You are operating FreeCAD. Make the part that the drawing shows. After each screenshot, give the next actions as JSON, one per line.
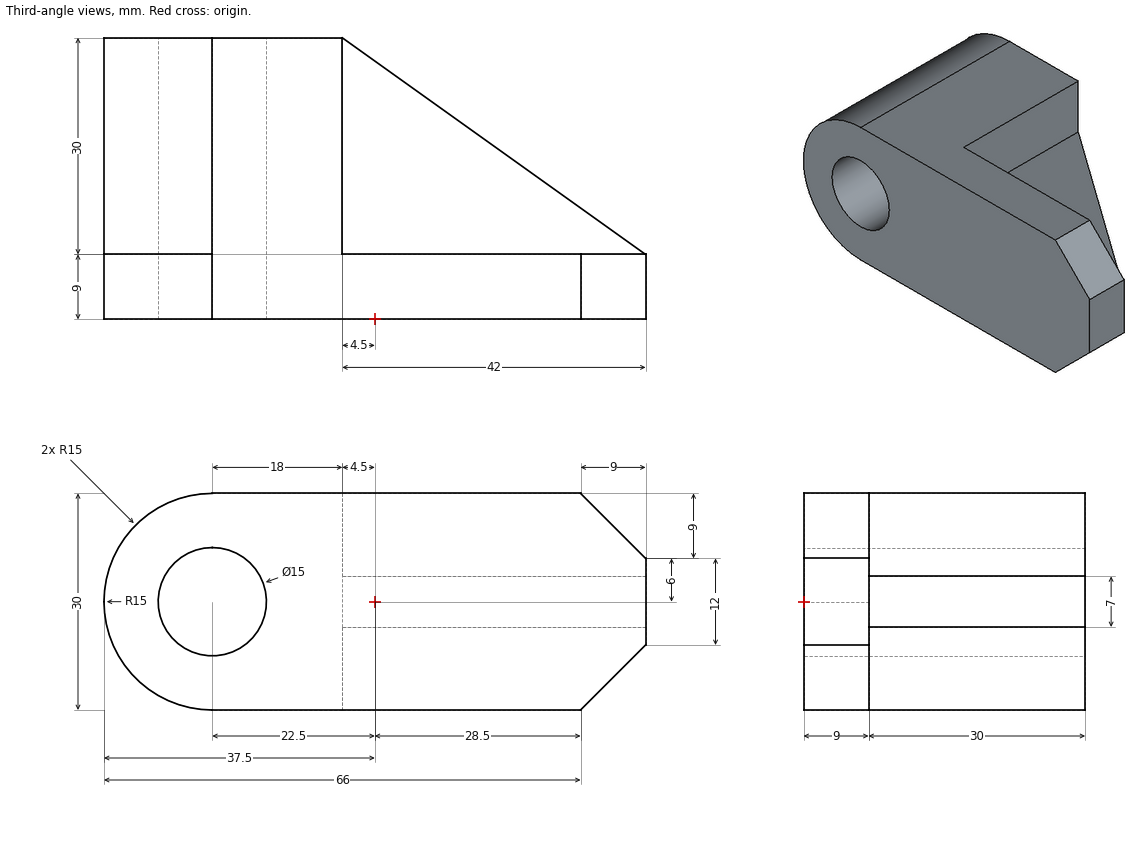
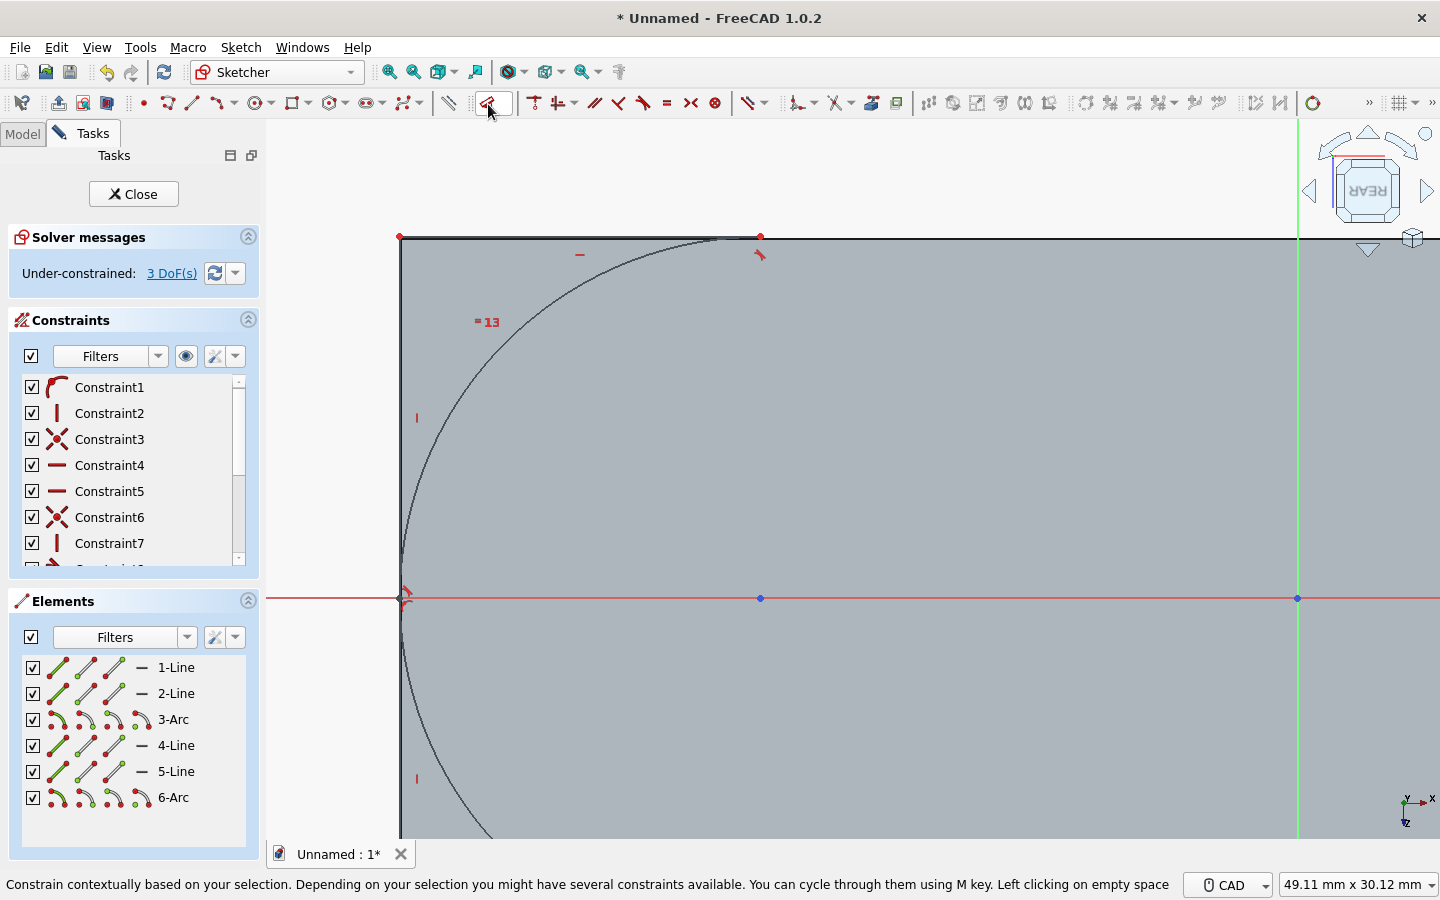
{"action": "left_click", "coordinate": [439, 762]}
{"action": "left_click", "coordinate": [421, 400]}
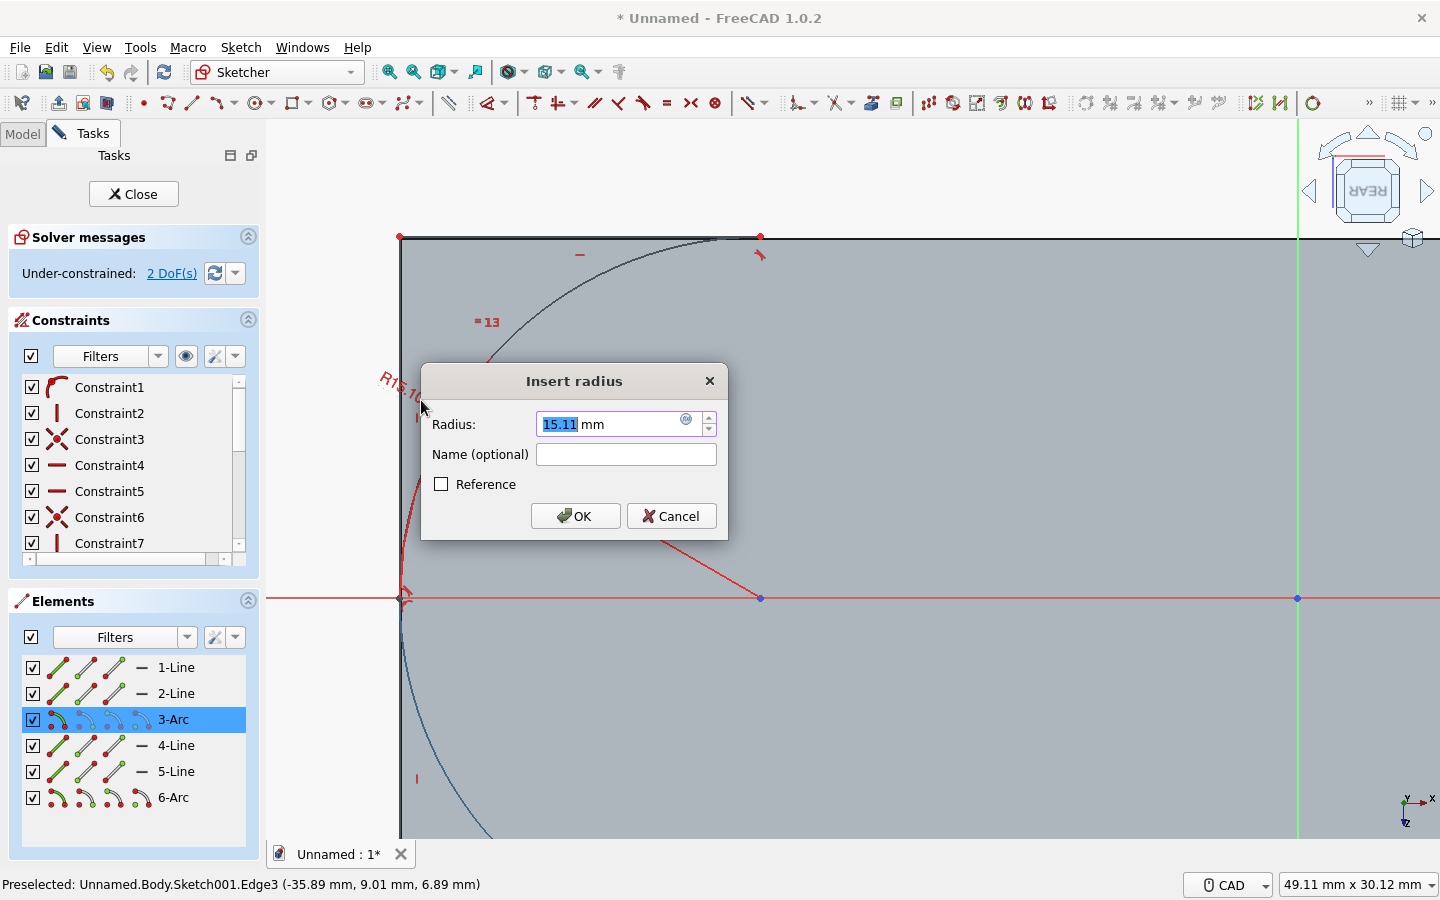
{"action": "type", "text": "15"}
{"action": "key", "text": "Return"}
{"action": "key", "text": "Escape"}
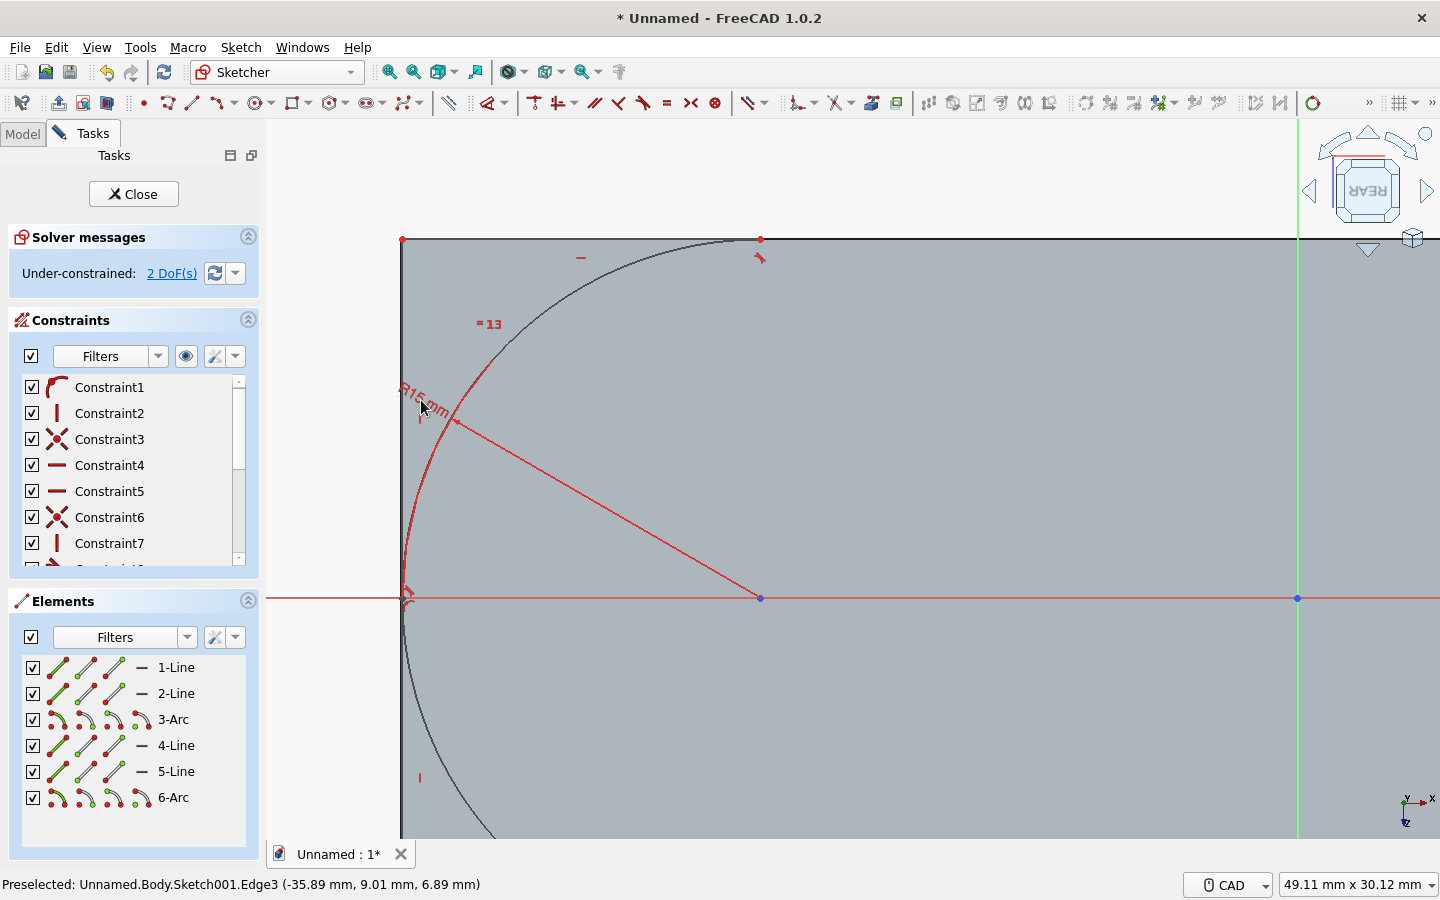
{"action": "left_click", "coordinate": [402, 598]}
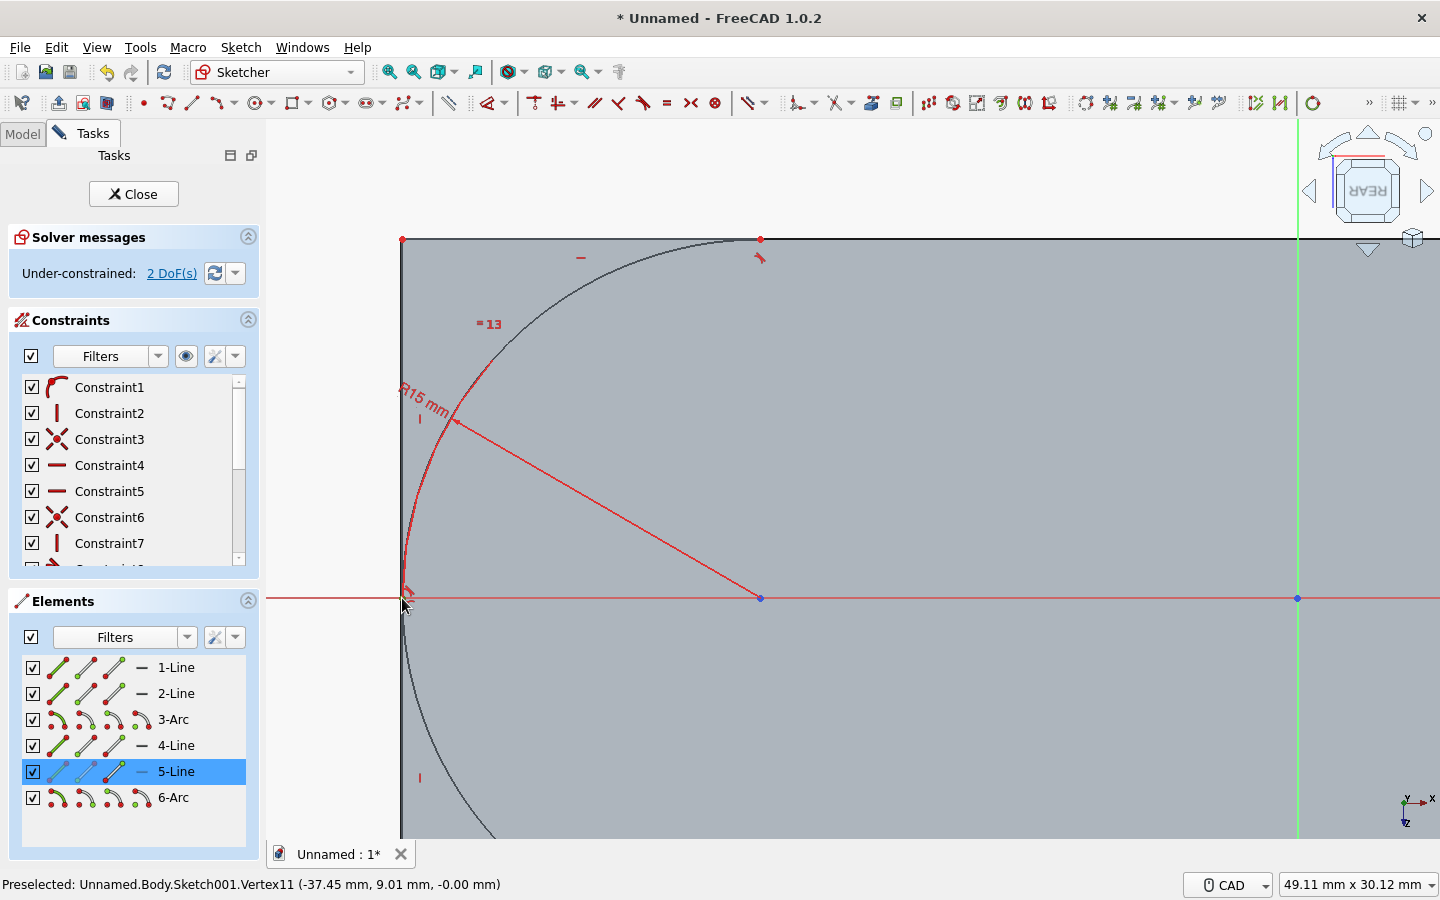
{"action": "left_click", "coordinate": [364, 598]}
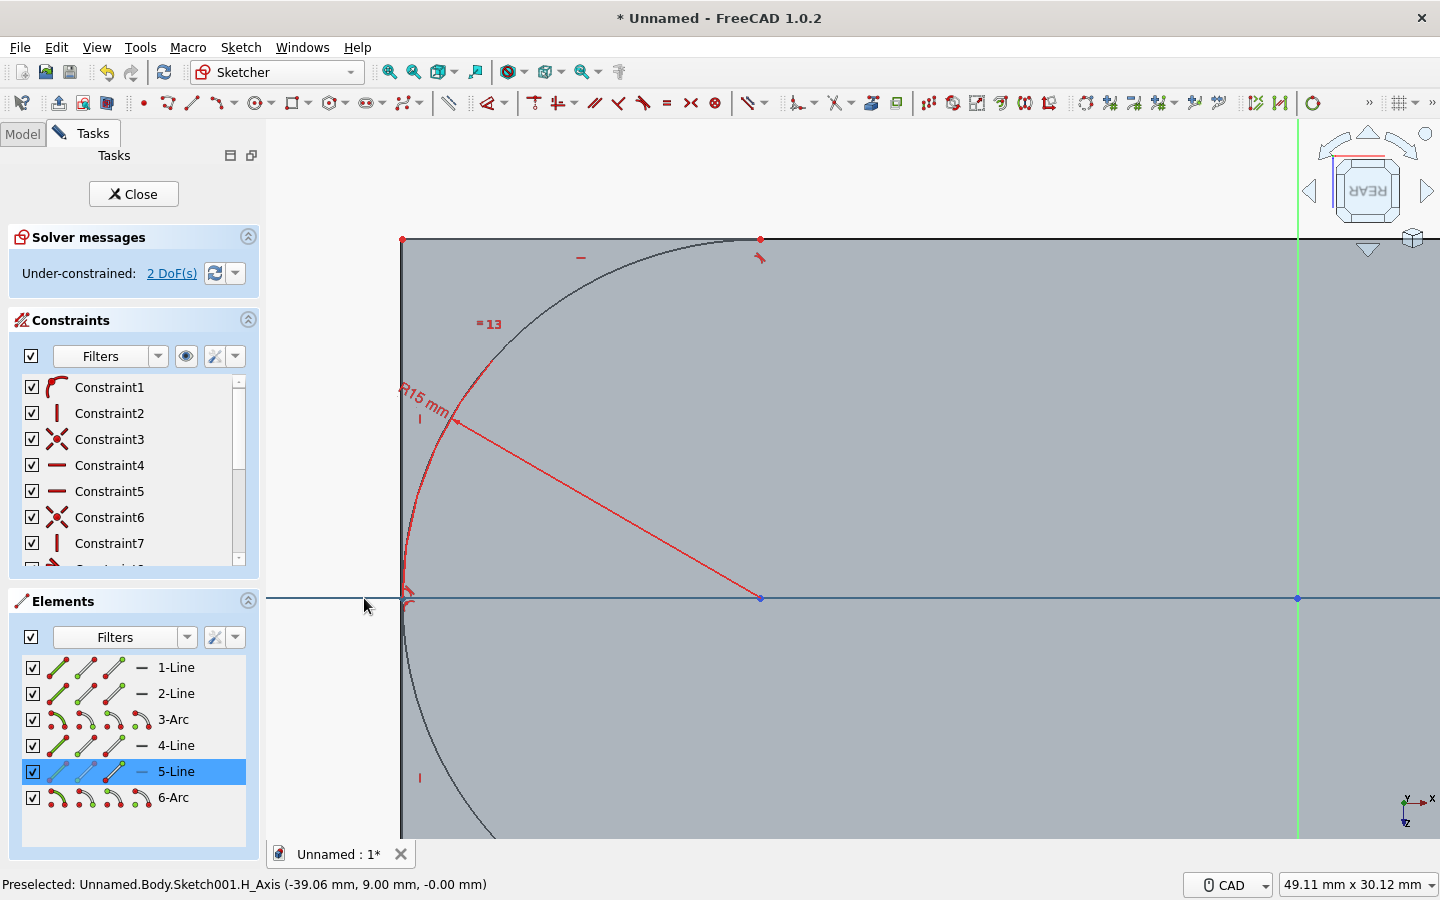
{"action": "left_click", "coordinate": [534, 104]}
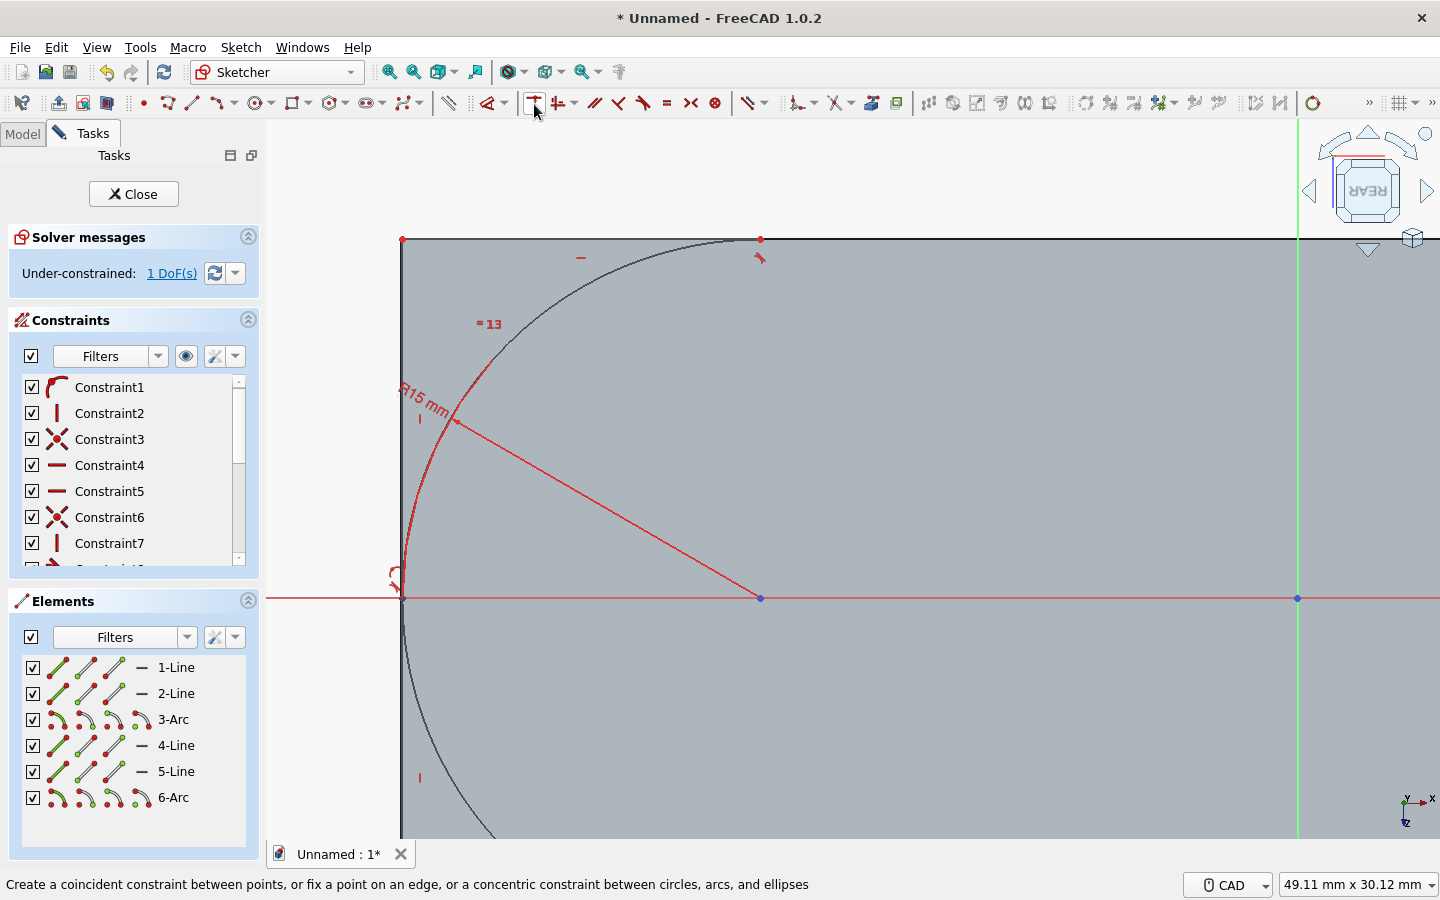
{"action": "left_click", "coordinate": [488, 104]}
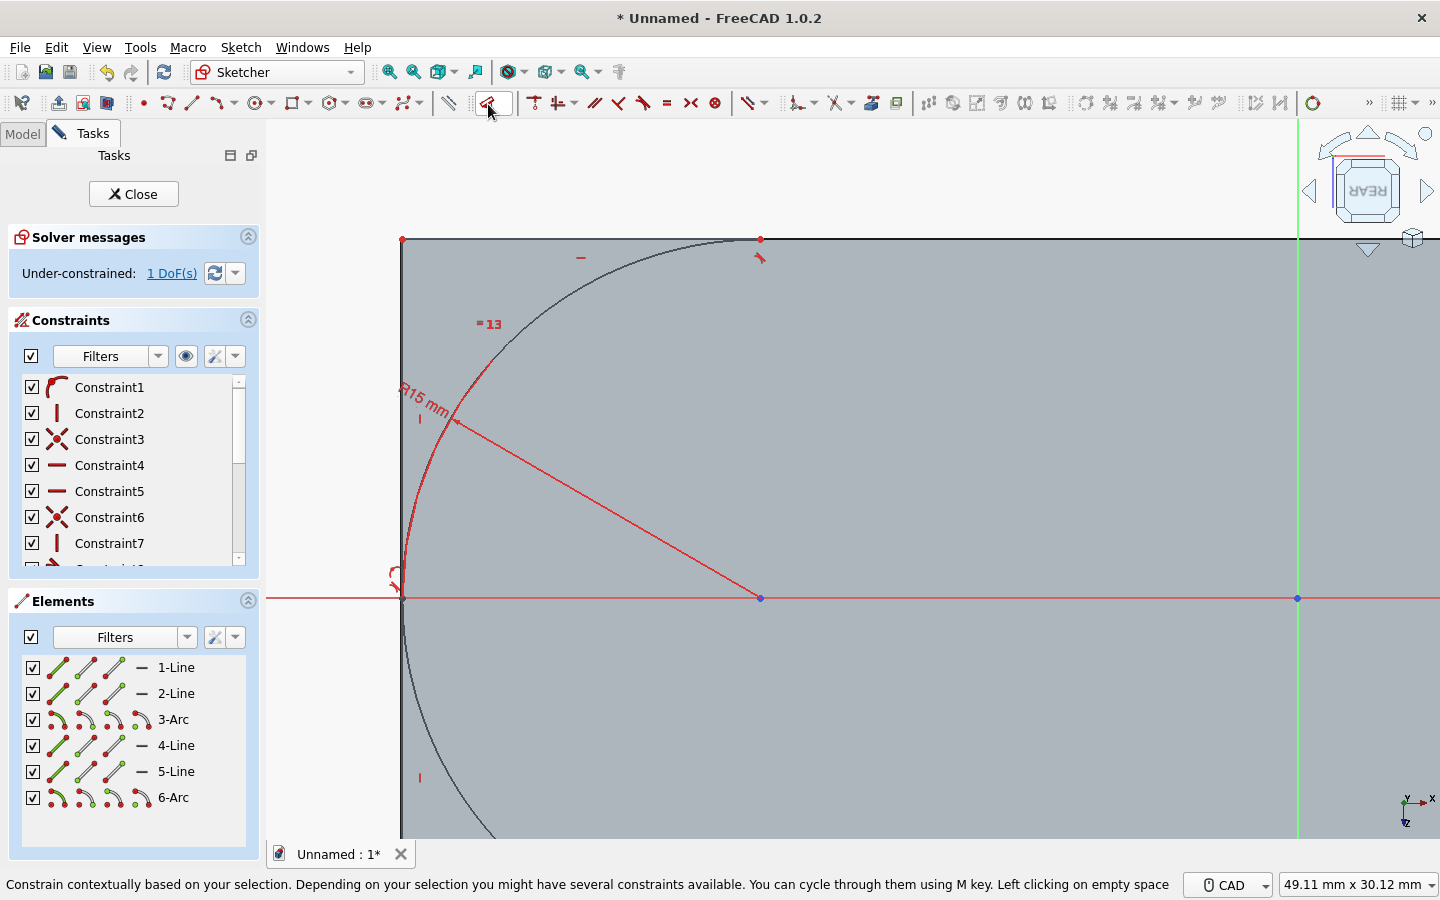
{"action": "left_click", "coordinate": [402, 598]}
{"action": "left_click", "coordinate": [839, 632]}